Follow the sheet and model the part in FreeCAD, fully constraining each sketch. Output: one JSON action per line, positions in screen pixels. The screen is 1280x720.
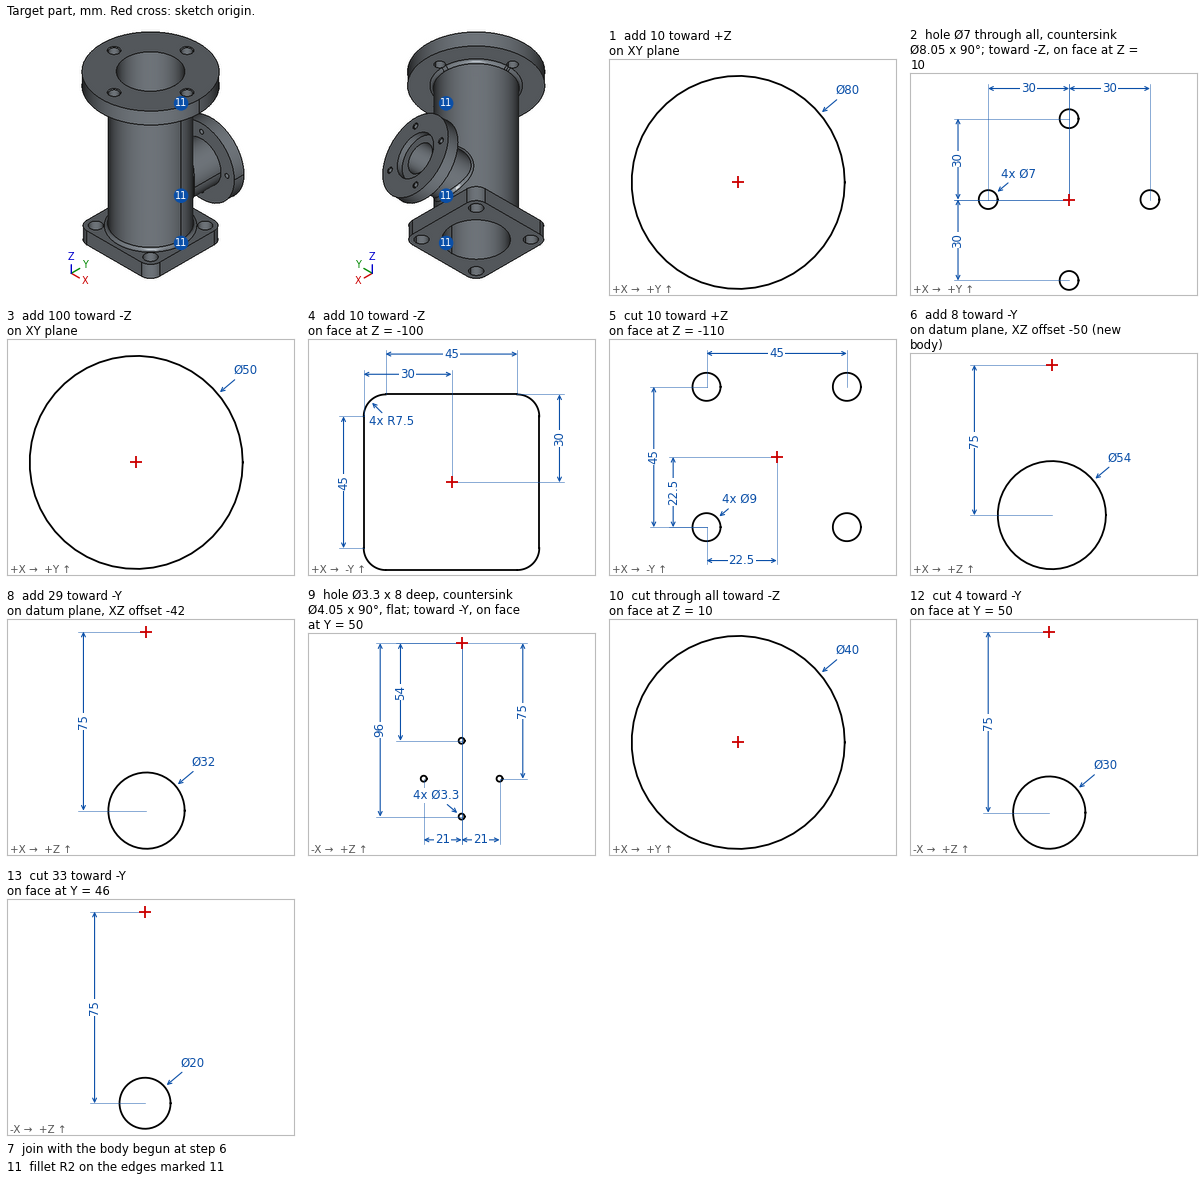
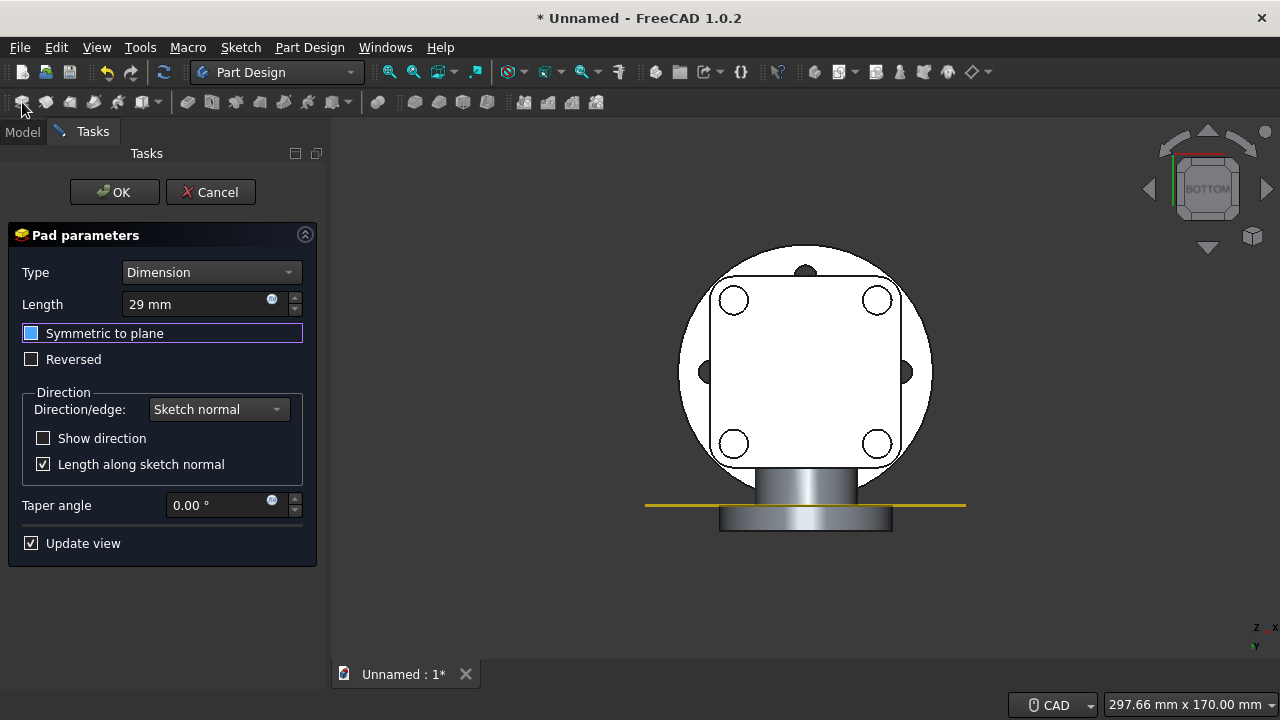
{"action": "left_click", "coordinate": [115, 192]}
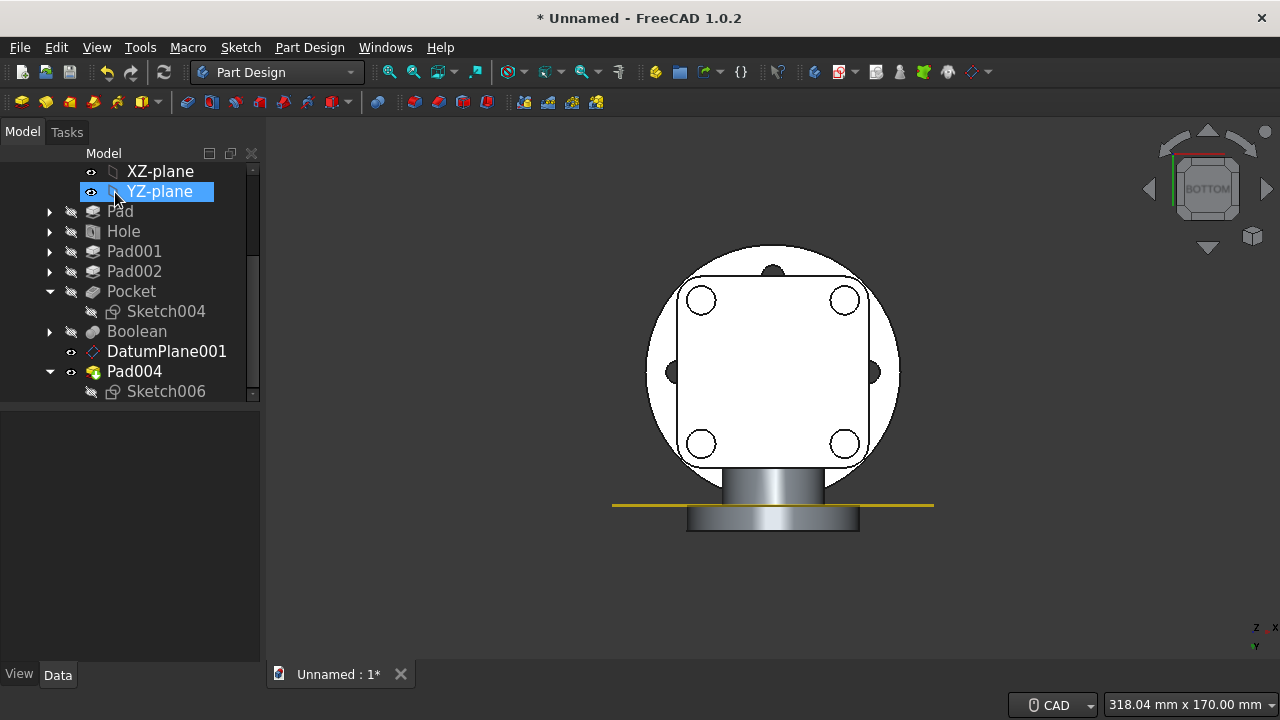
{"action": "left_click", "coordinate": [116, 352]}
{"action": "key", "text": "space"}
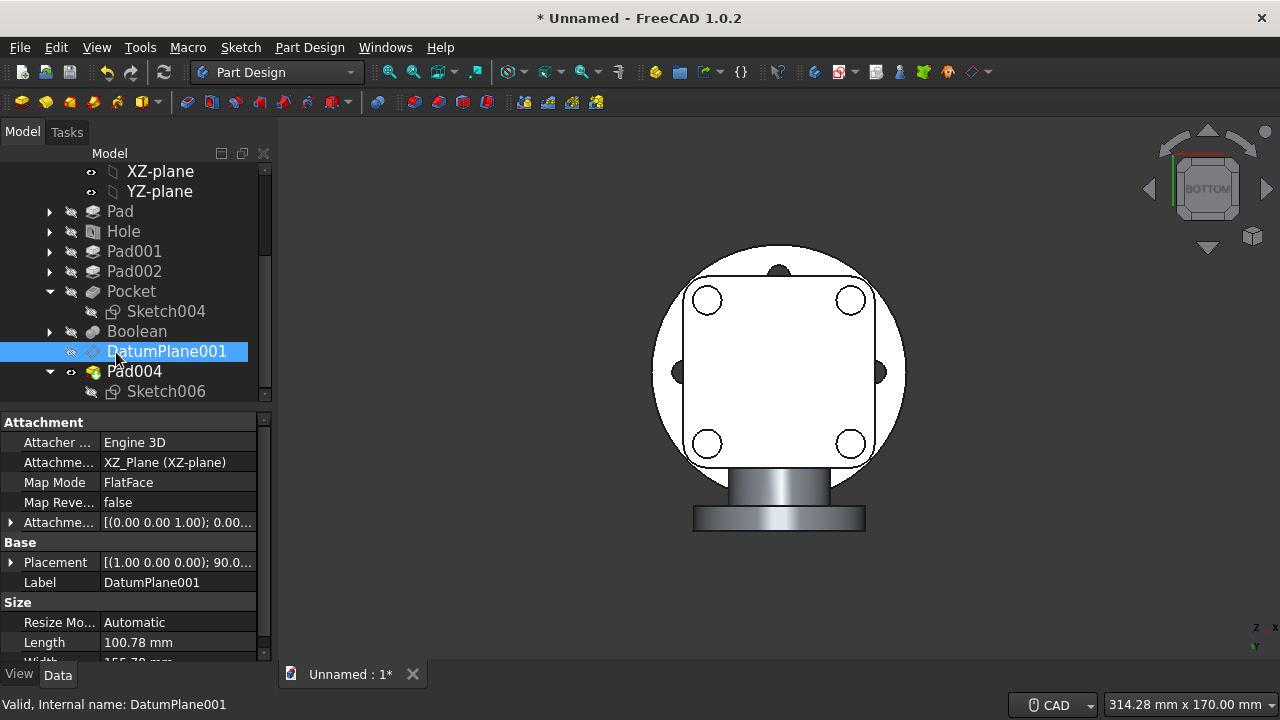
{"action": "key", "text": "4"}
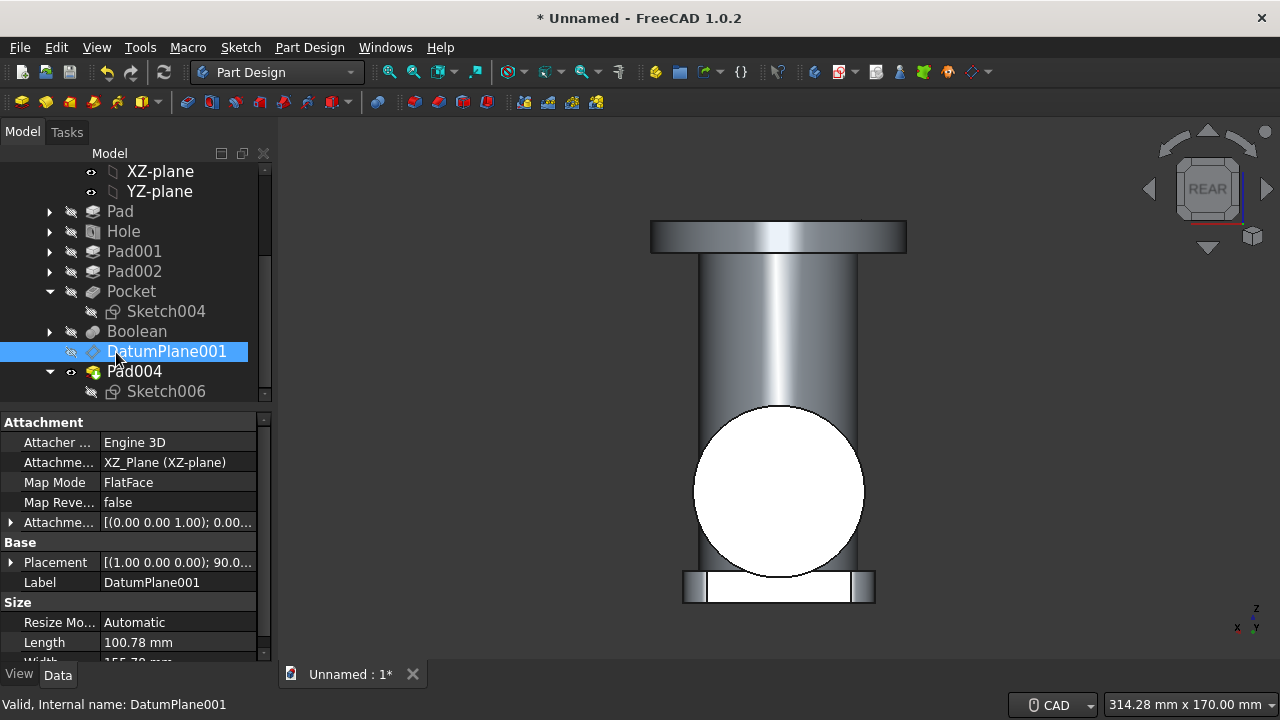
{"action": "left_click", "coordinate": [779, 491]}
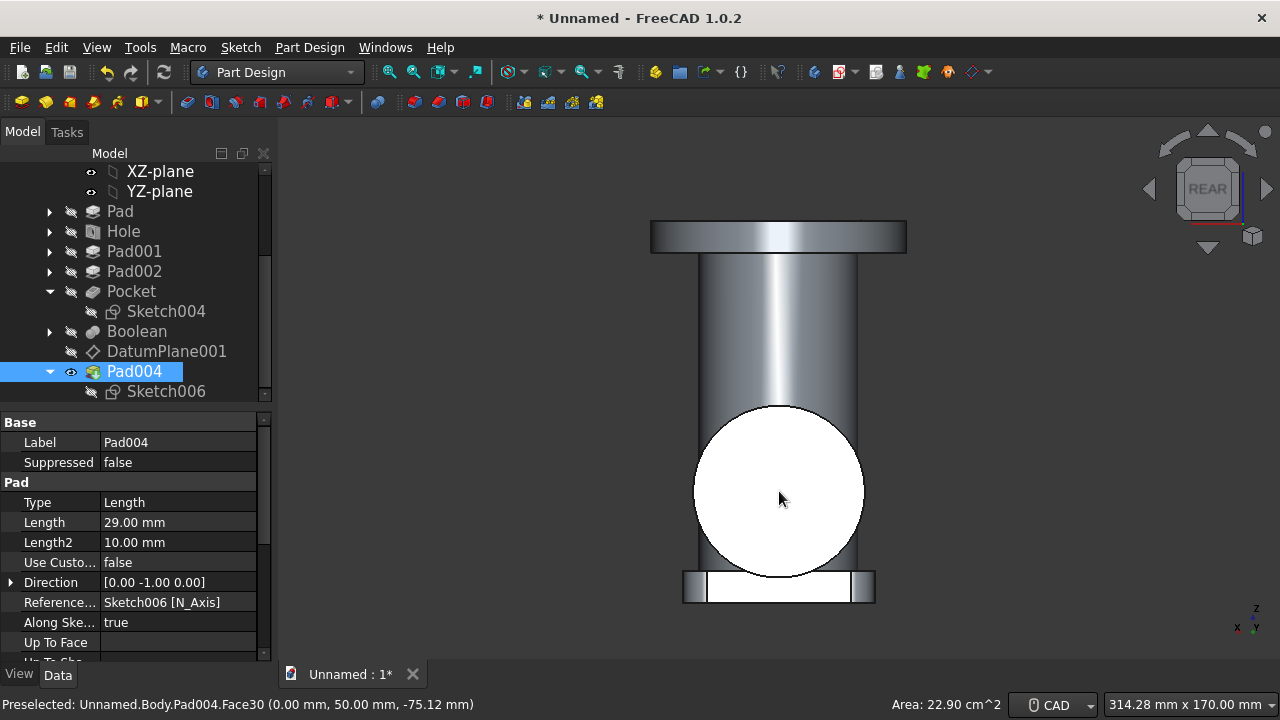
{"action": "left_click", "coordinate": [840, 72]}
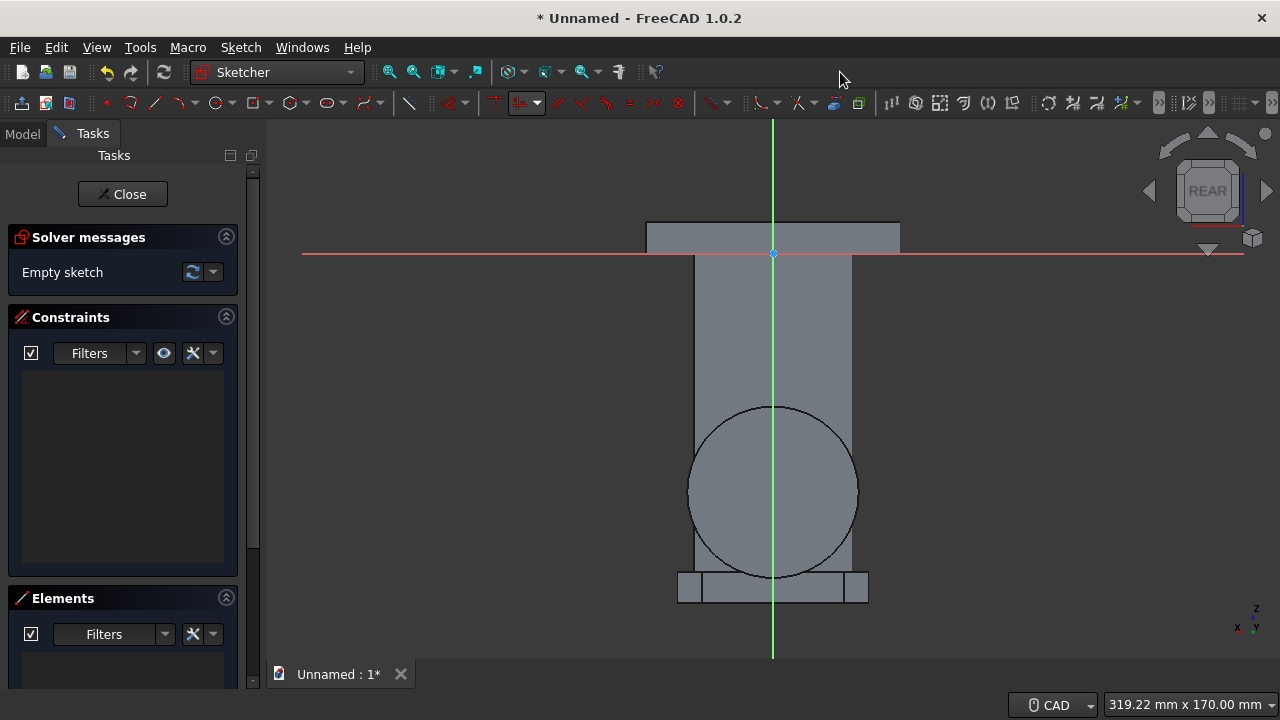
{"action": "left_click", "coordinate": [216, 104]}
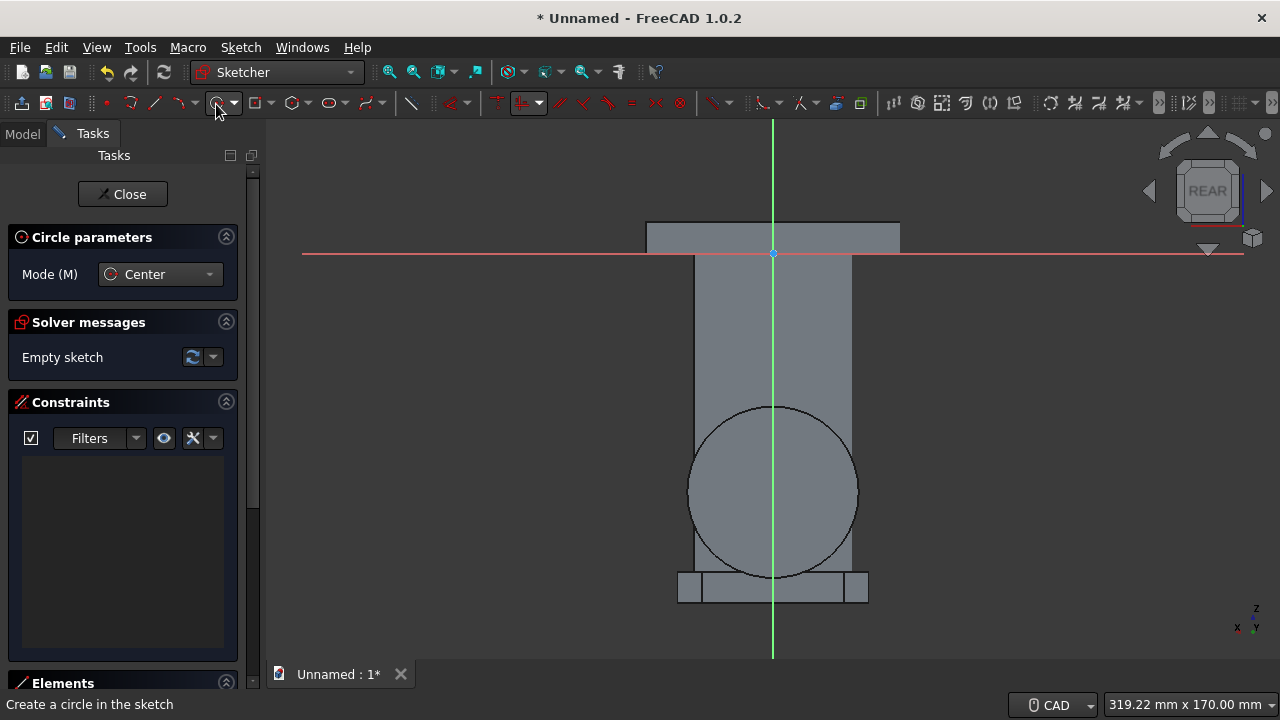
{"action": "scroll", "coordinate": [773, 559], "scroll_direction": "up", "scroll_amount": 8}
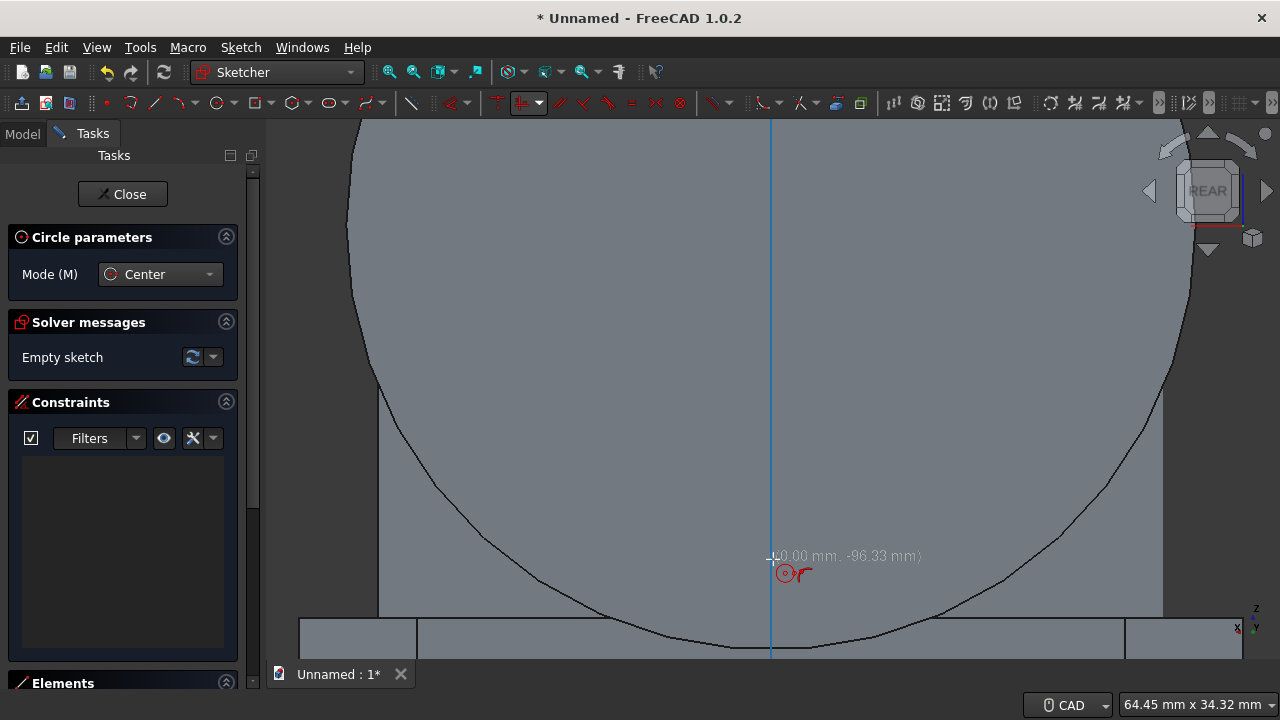
{"action": "scroll", "coordinate": [688, 535], "scroll_direction": "down", "scroll_amount": 8}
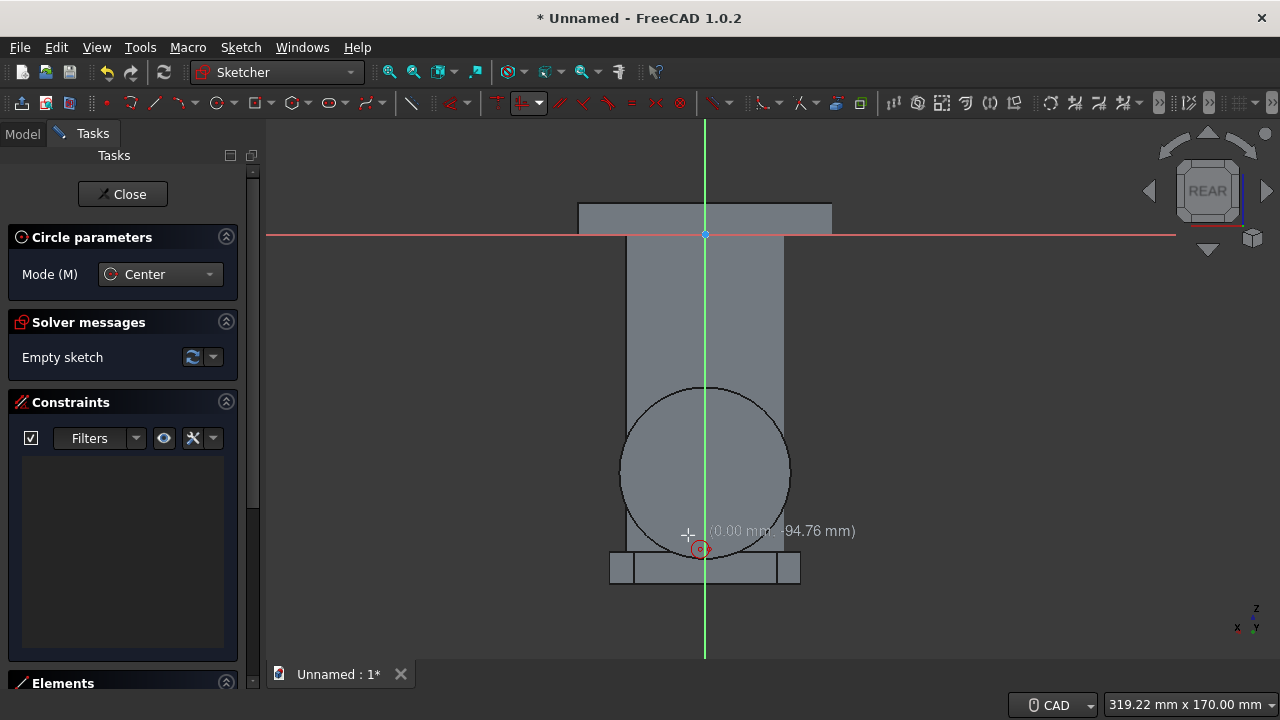
{"action": "left_click", "coordinate": [705, 540]}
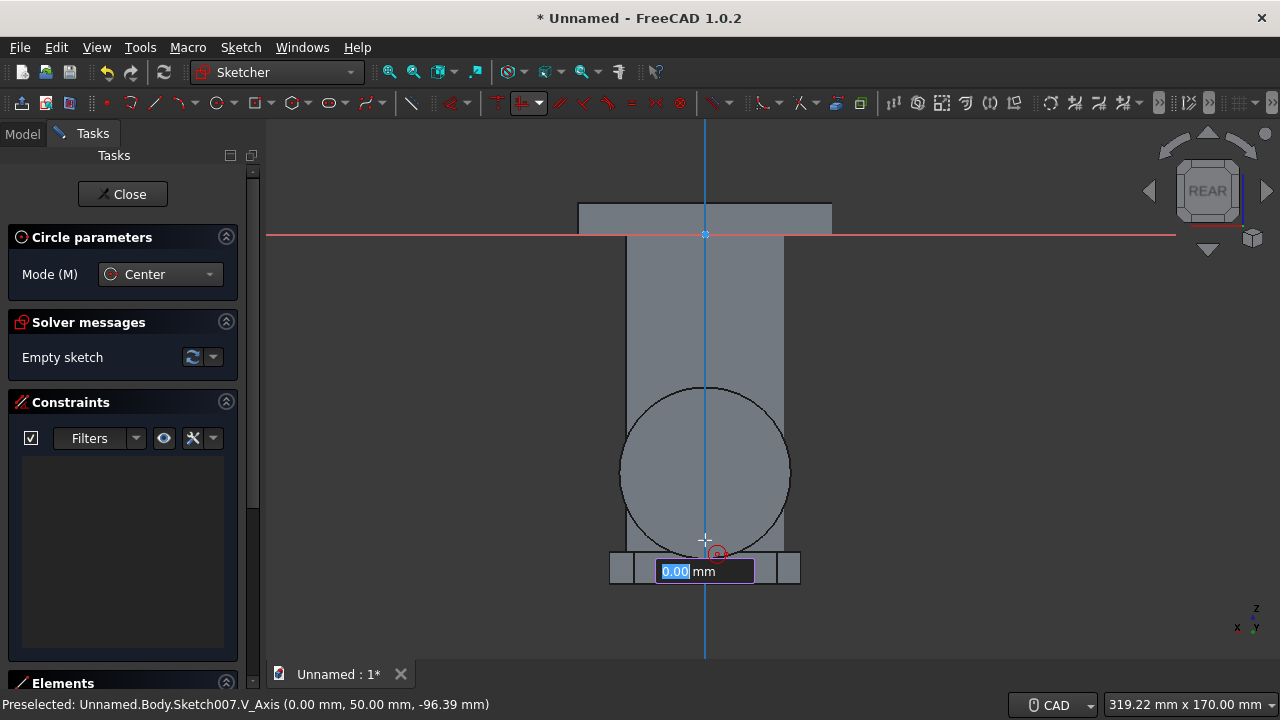
{"action": "scroll", "coordinate": [710, 538], "scroll_direction": "up", "scroll_amount": 6}
{"action": "mouse_move", "coordinate": [709, 536]}